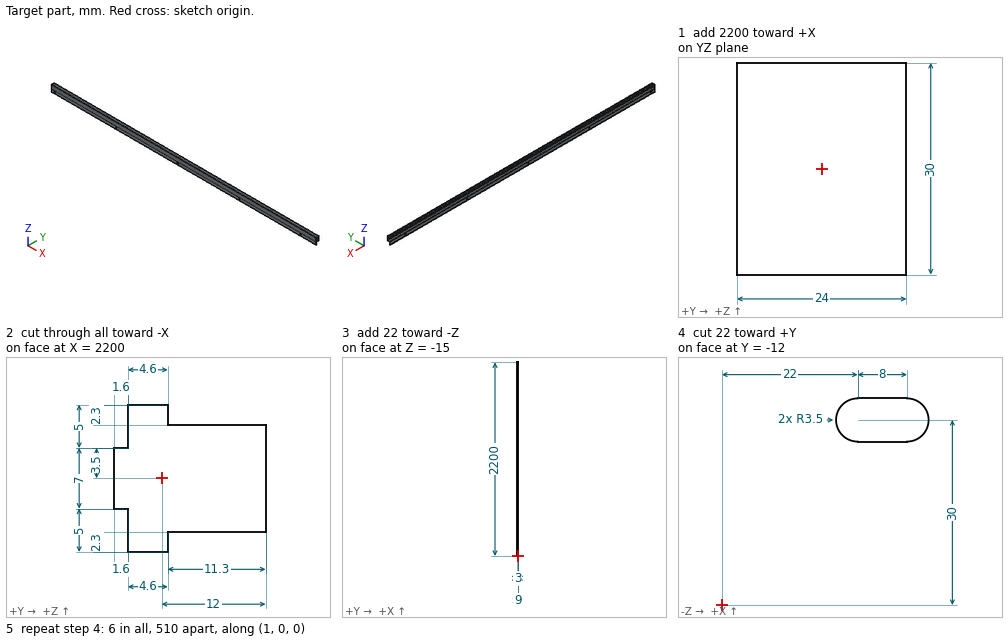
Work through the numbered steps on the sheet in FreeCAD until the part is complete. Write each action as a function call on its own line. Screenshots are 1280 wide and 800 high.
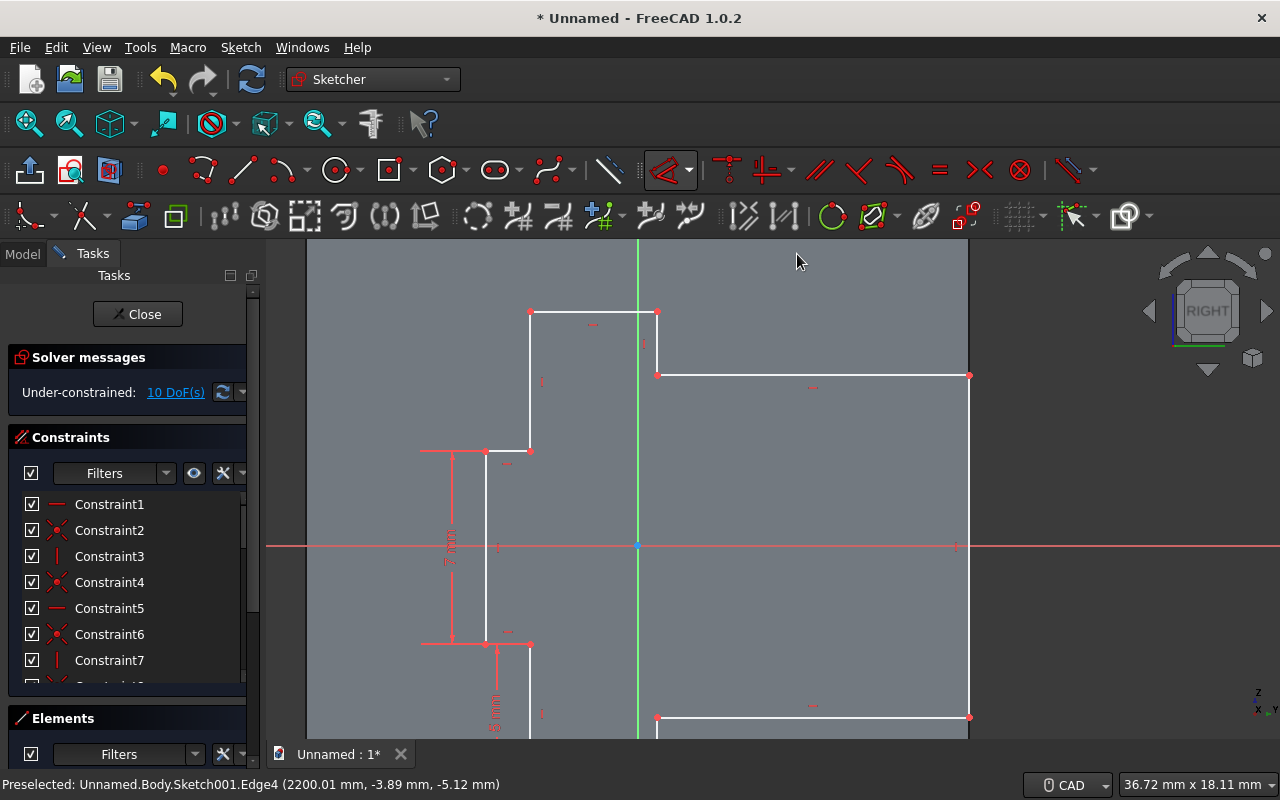
click(530, 354)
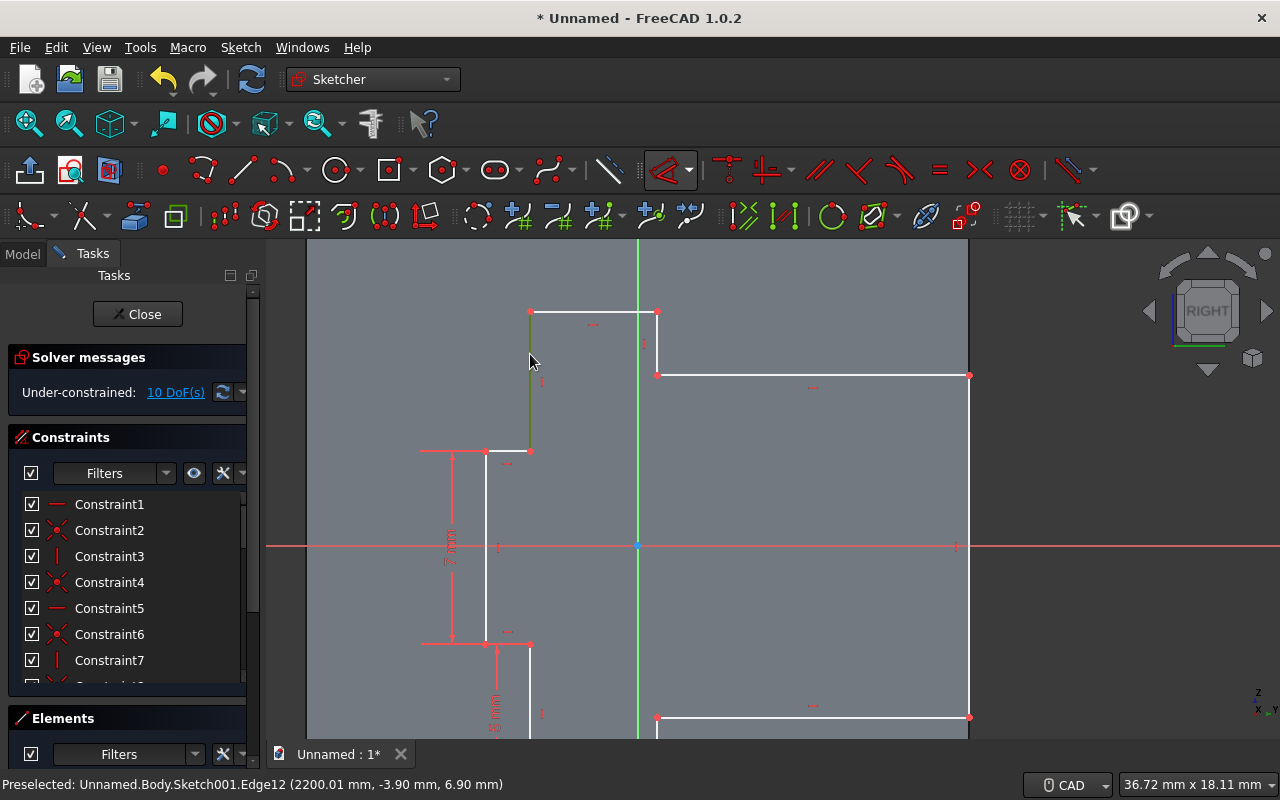
click(692, 170)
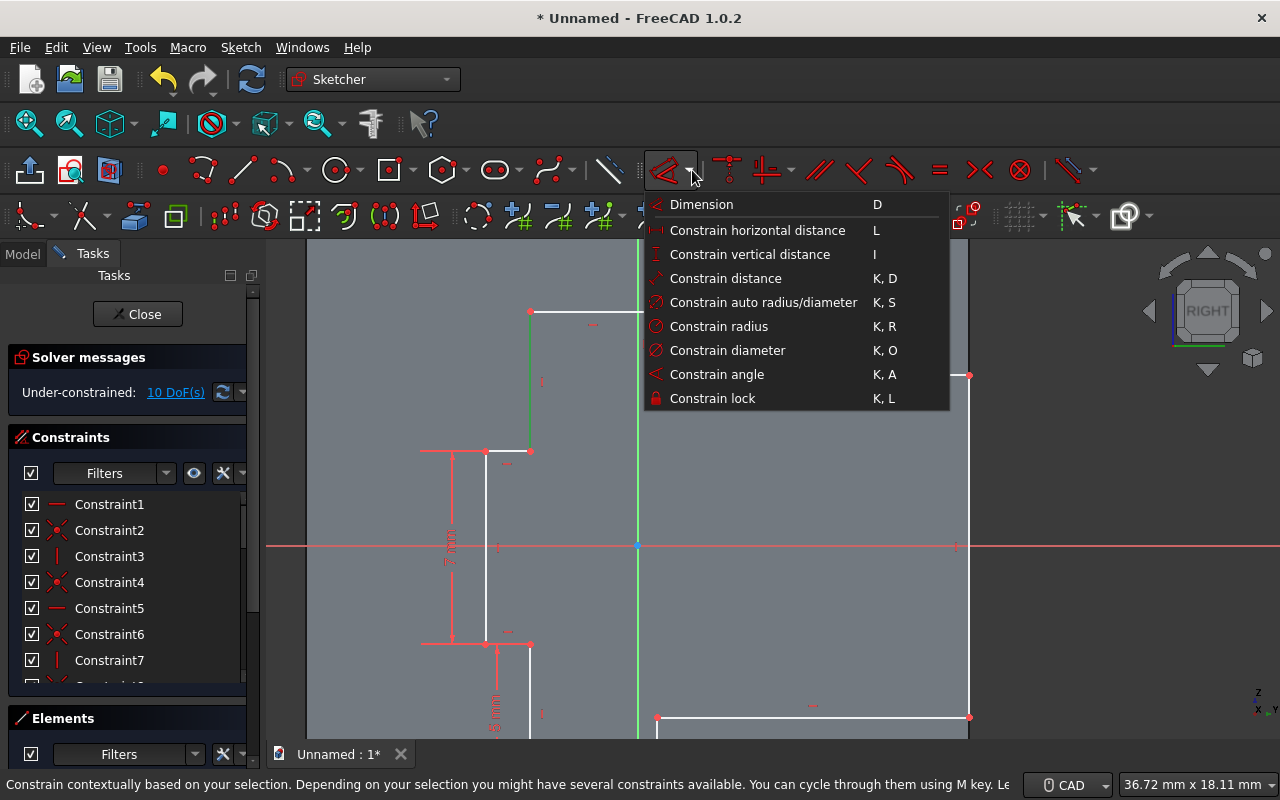
click(797, 254)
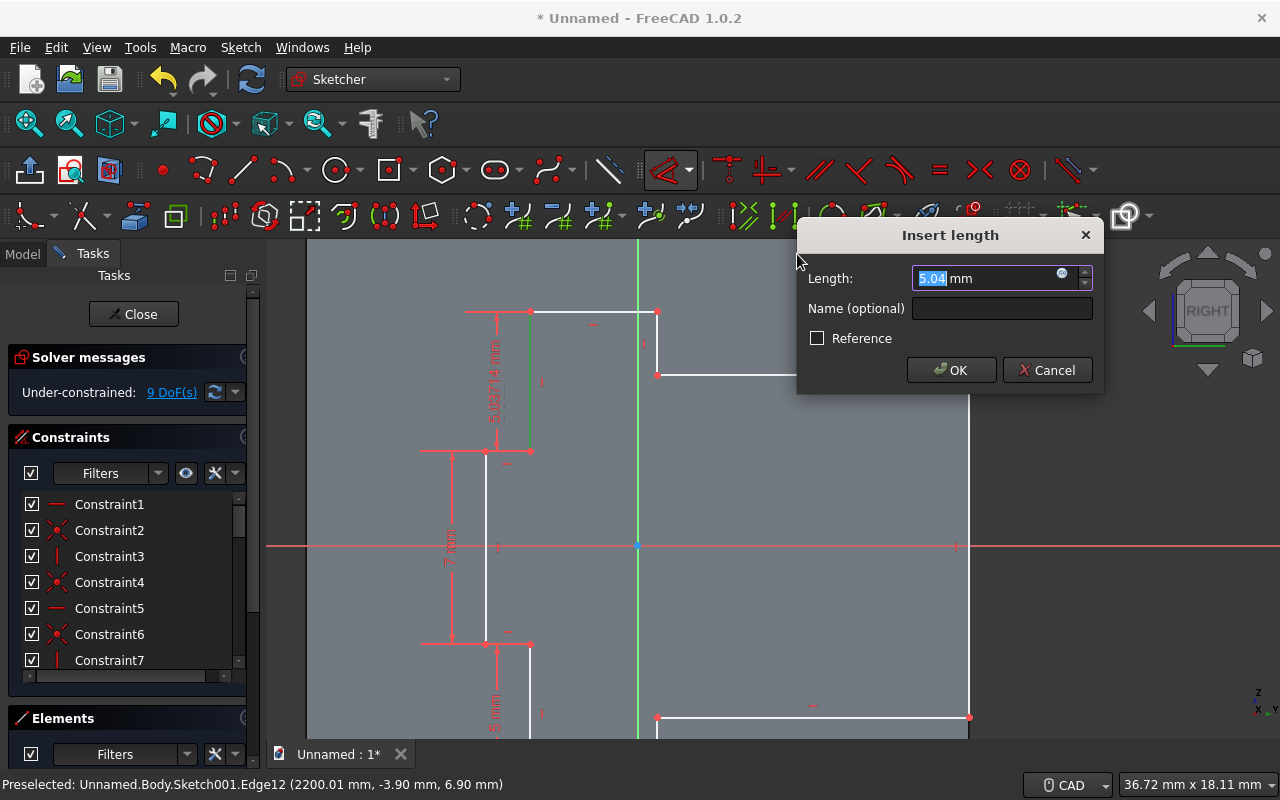
text(5)
key(Return)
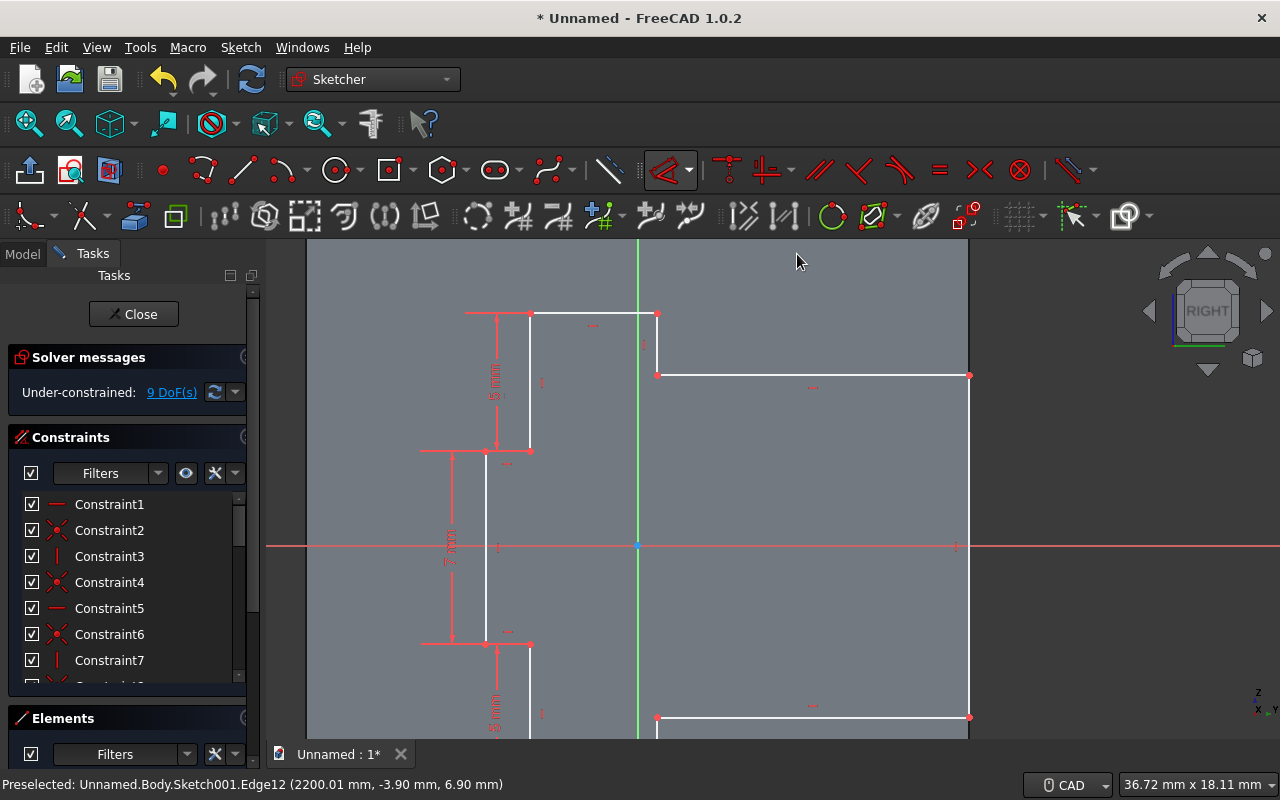
click(517, 451)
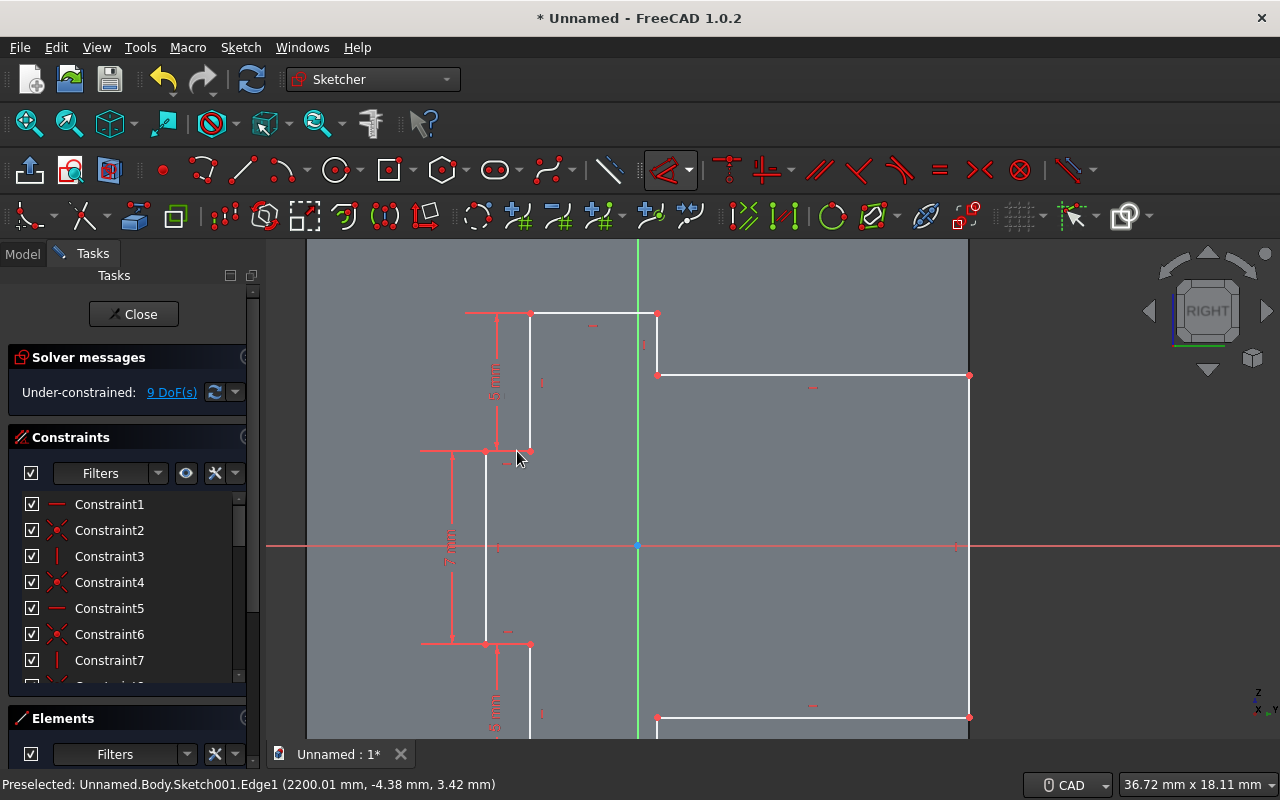
click(692, 170)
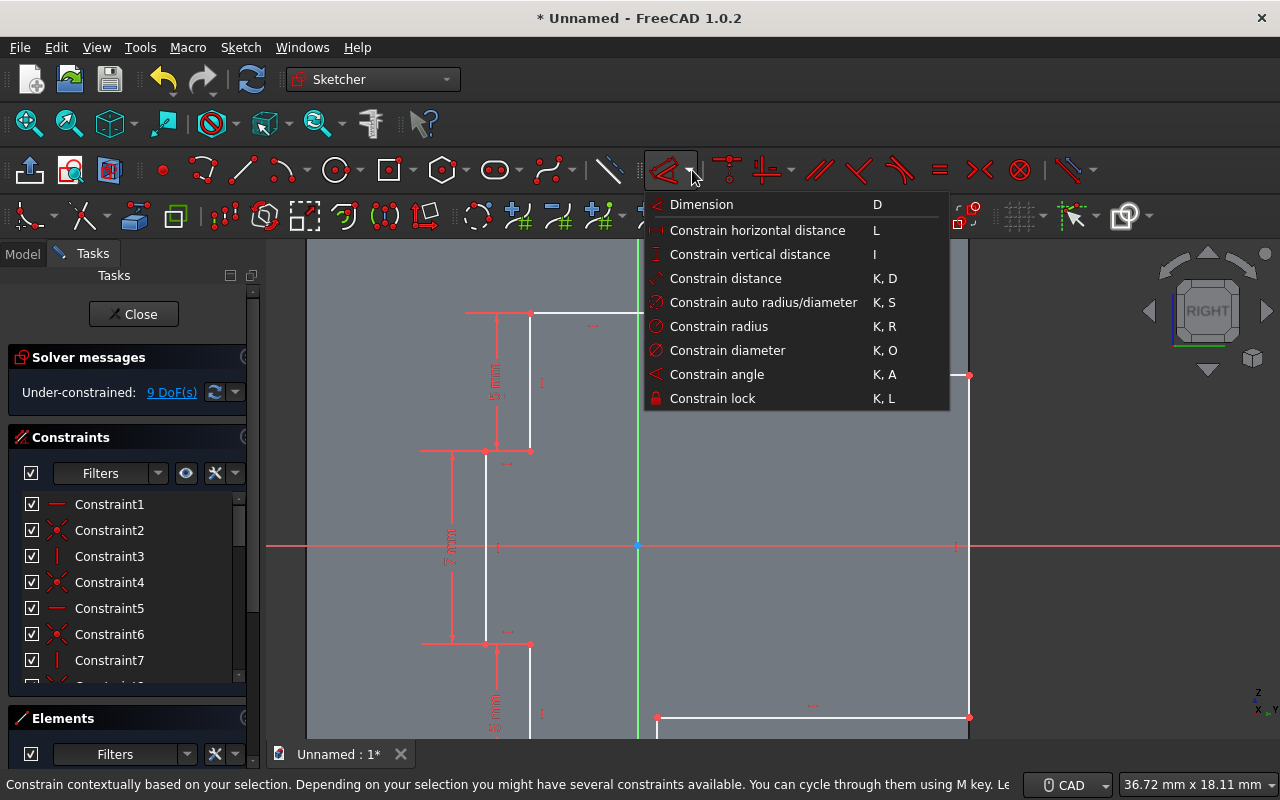
click(797, 230)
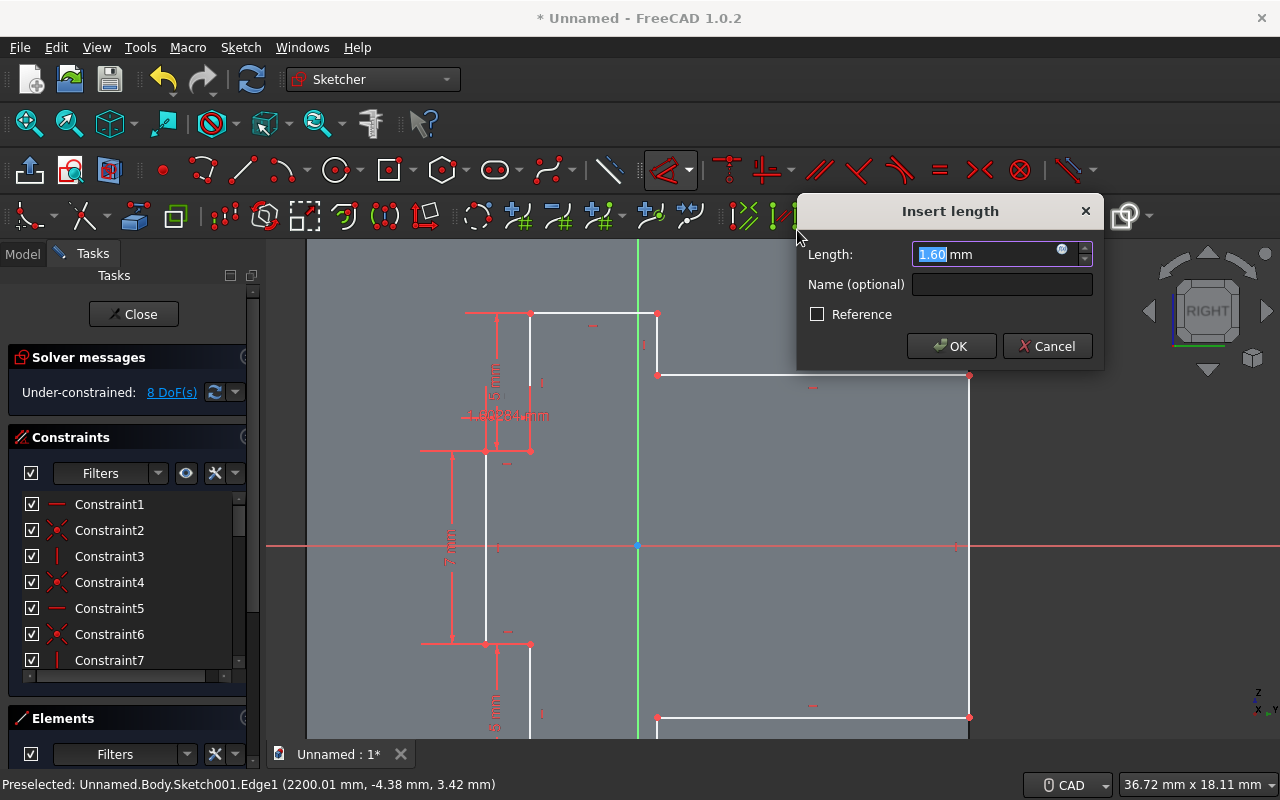
text(1.6)
key(Return)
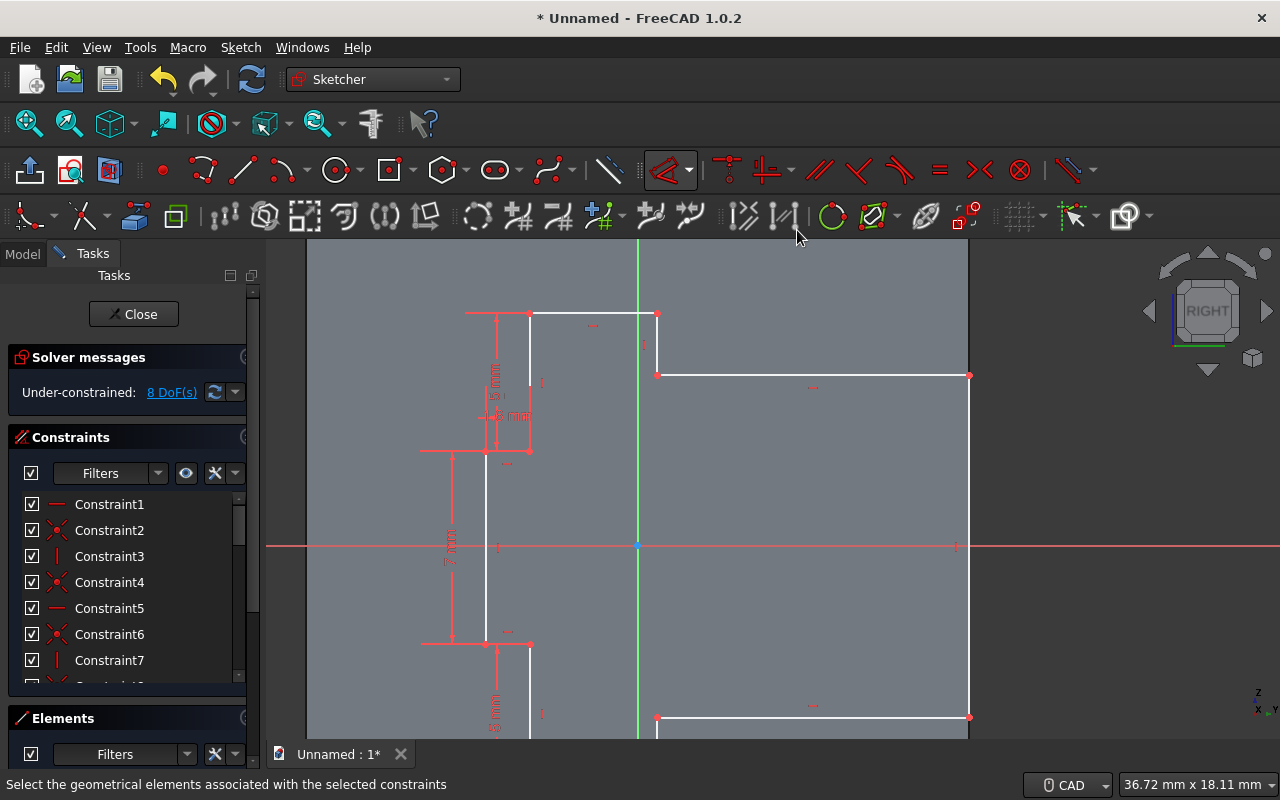
click(499, 644)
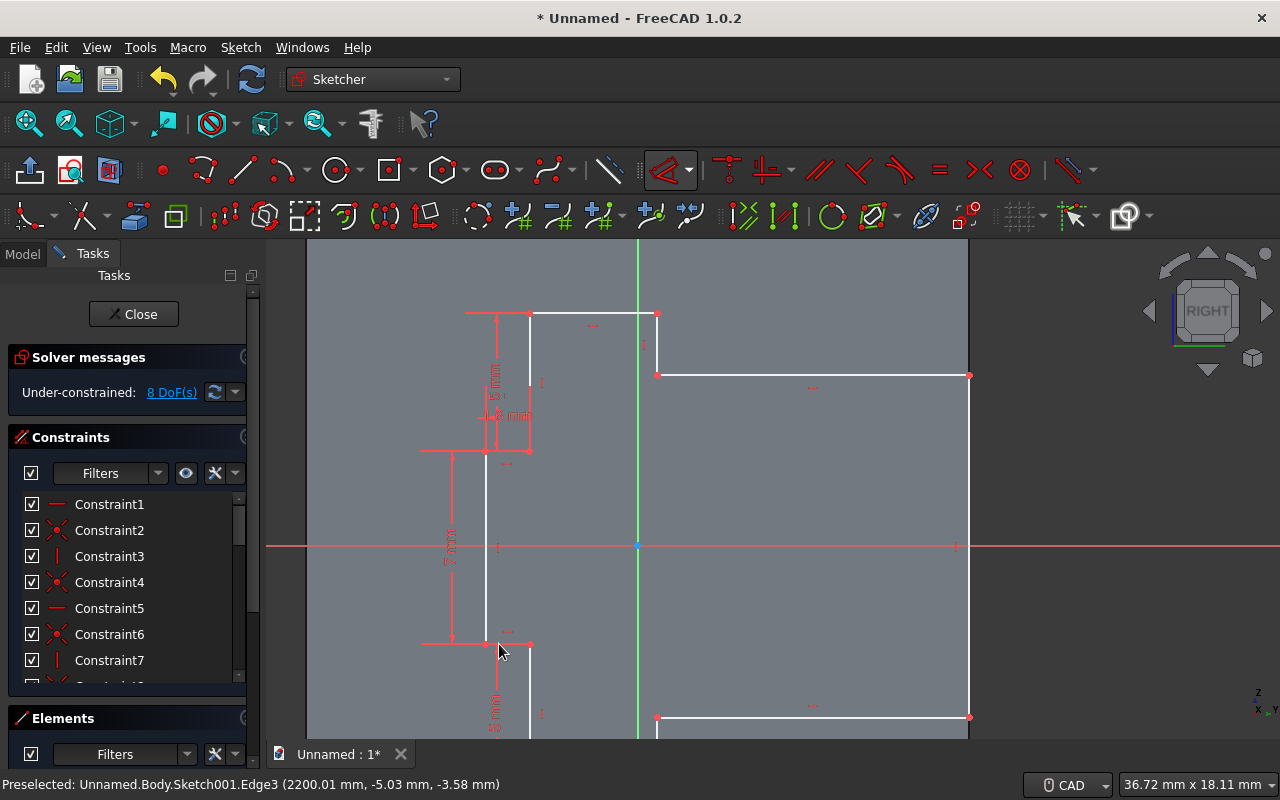
click(692, 170)